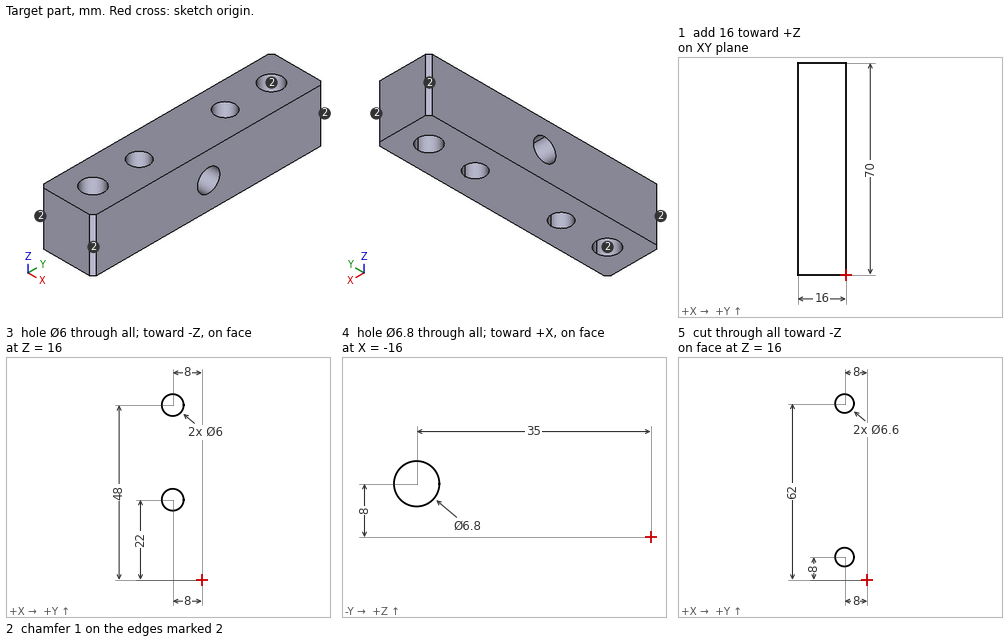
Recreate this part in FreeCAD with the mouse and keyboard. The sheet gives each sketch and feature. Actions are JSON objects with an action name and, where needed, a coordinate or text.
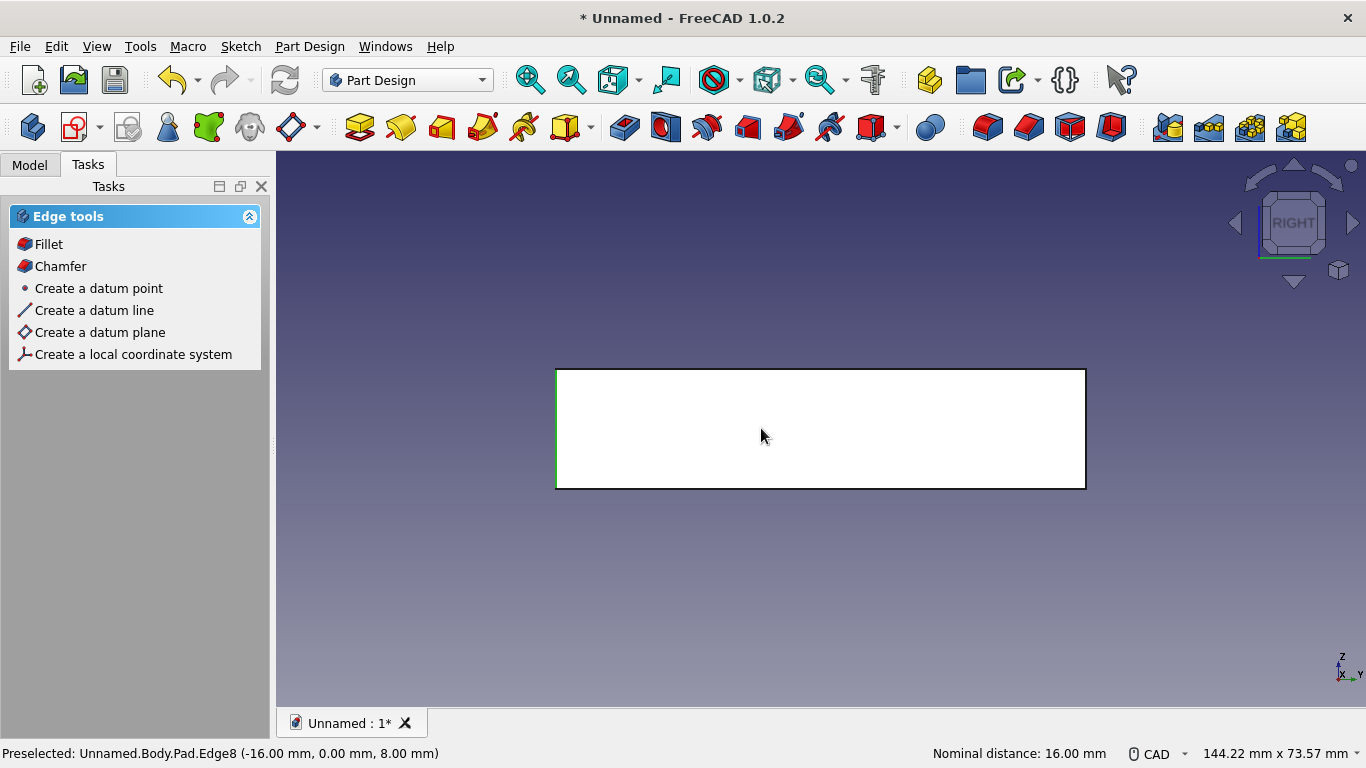
{"action": "left_click", "coordinate": [1086, 428], "text": "ctrl"}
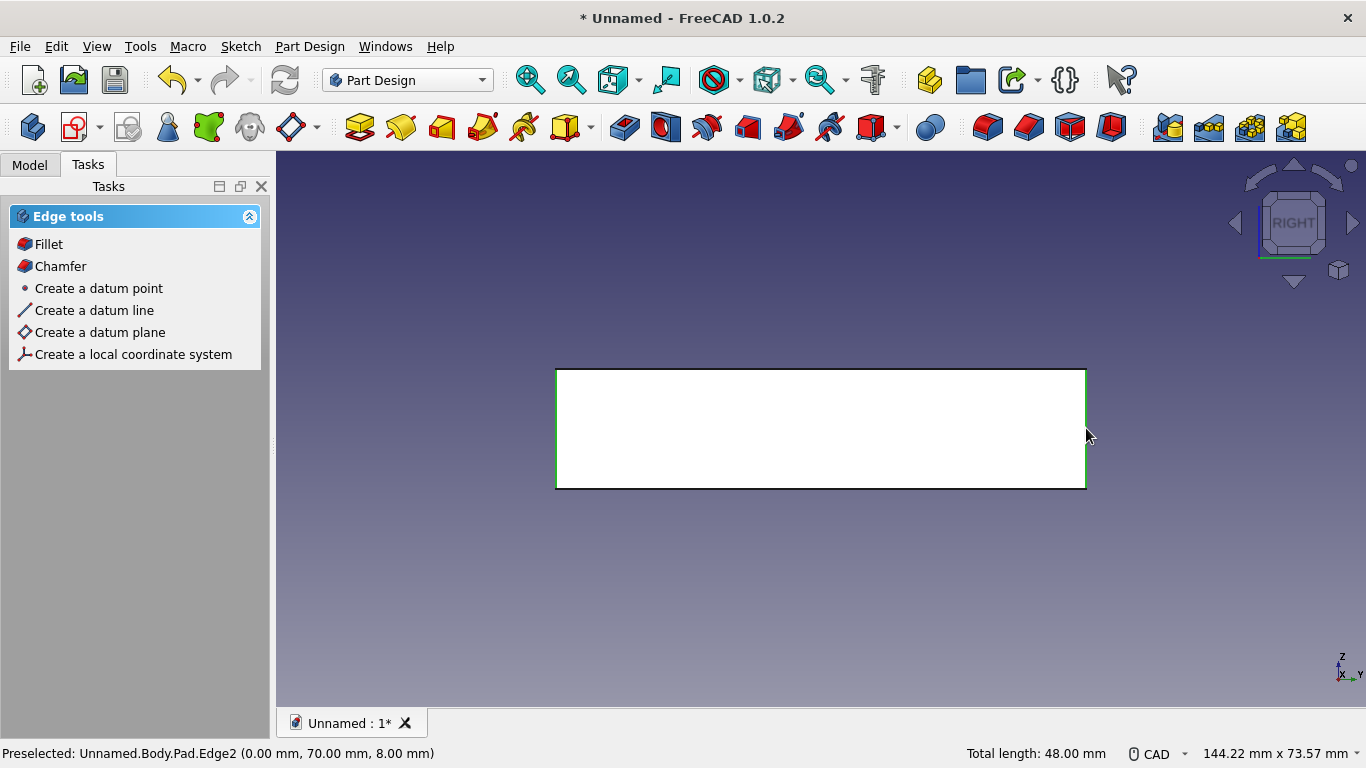
{"action": "key", "text": "5"}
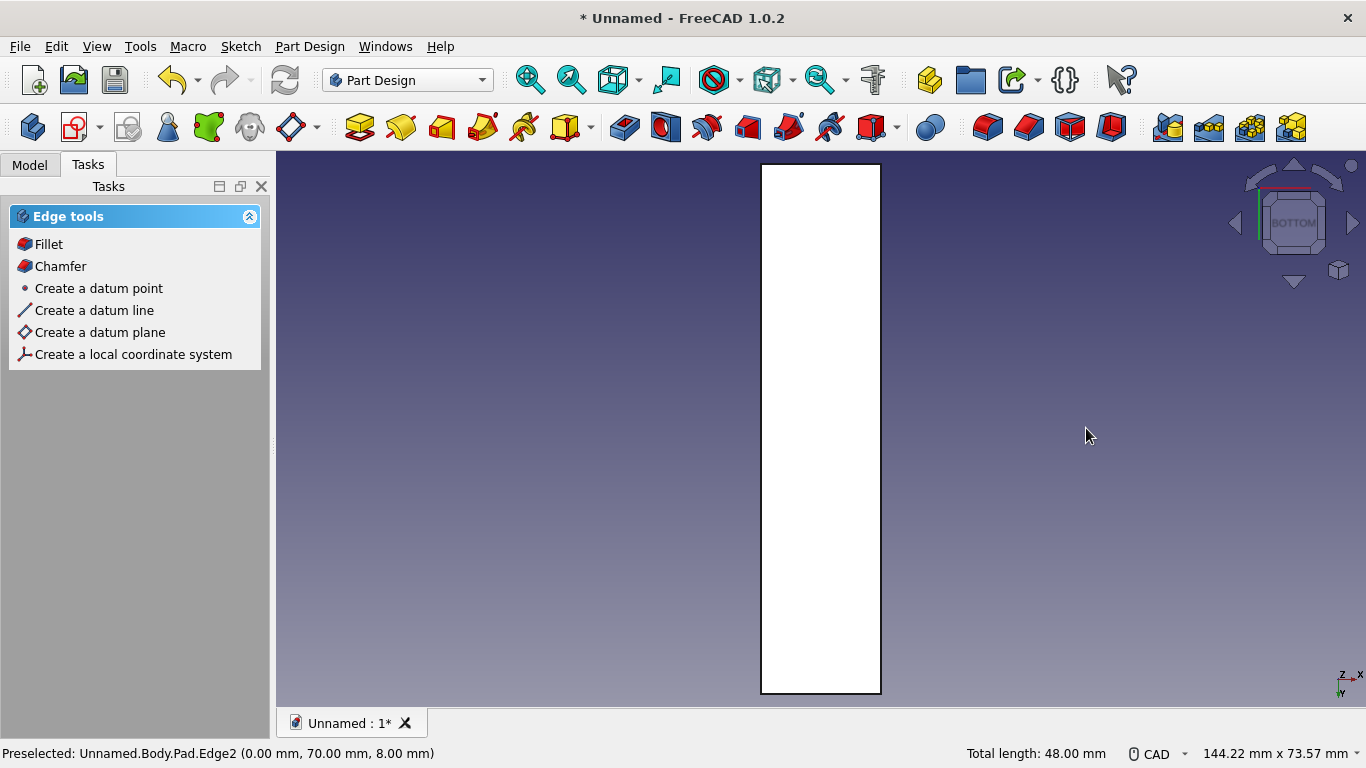
{"action": "key", "text": "4"}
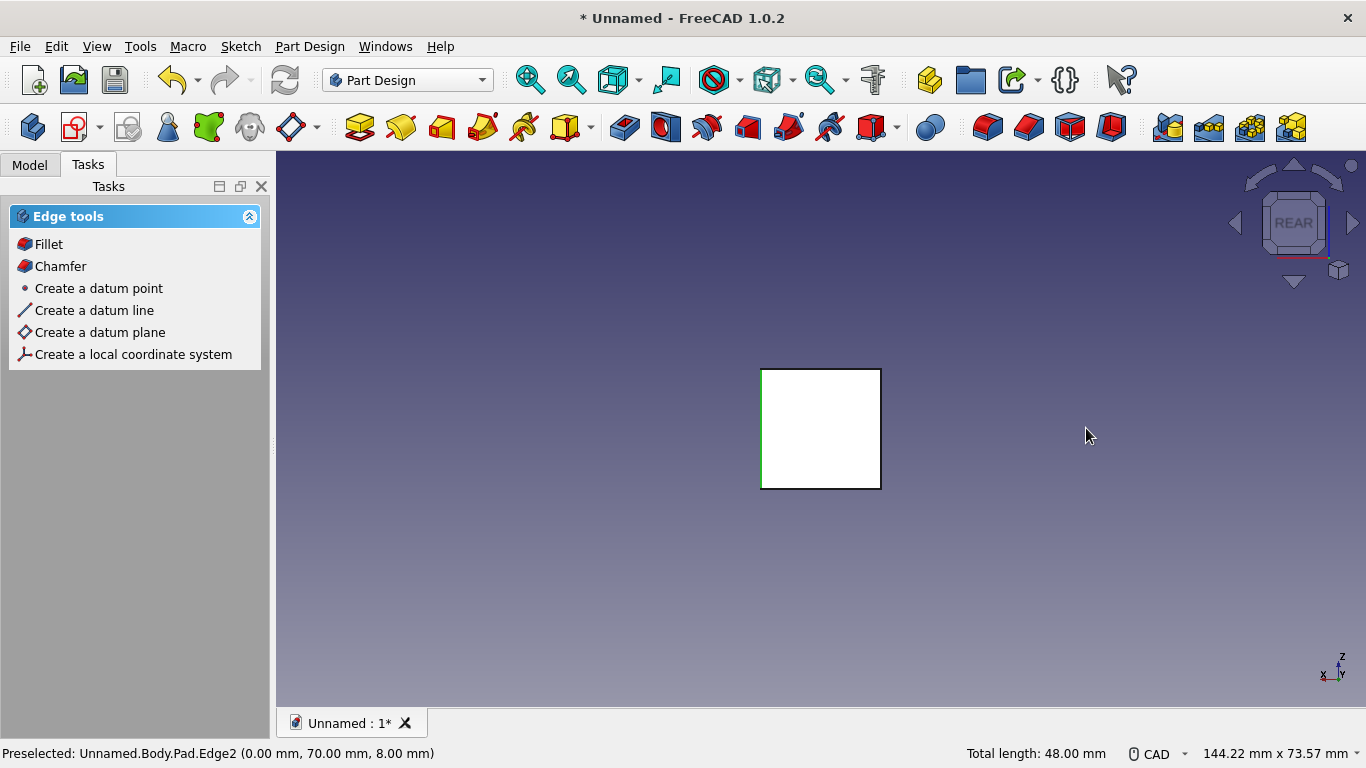
{"action": "left_click", "coordinate": [531, 80]}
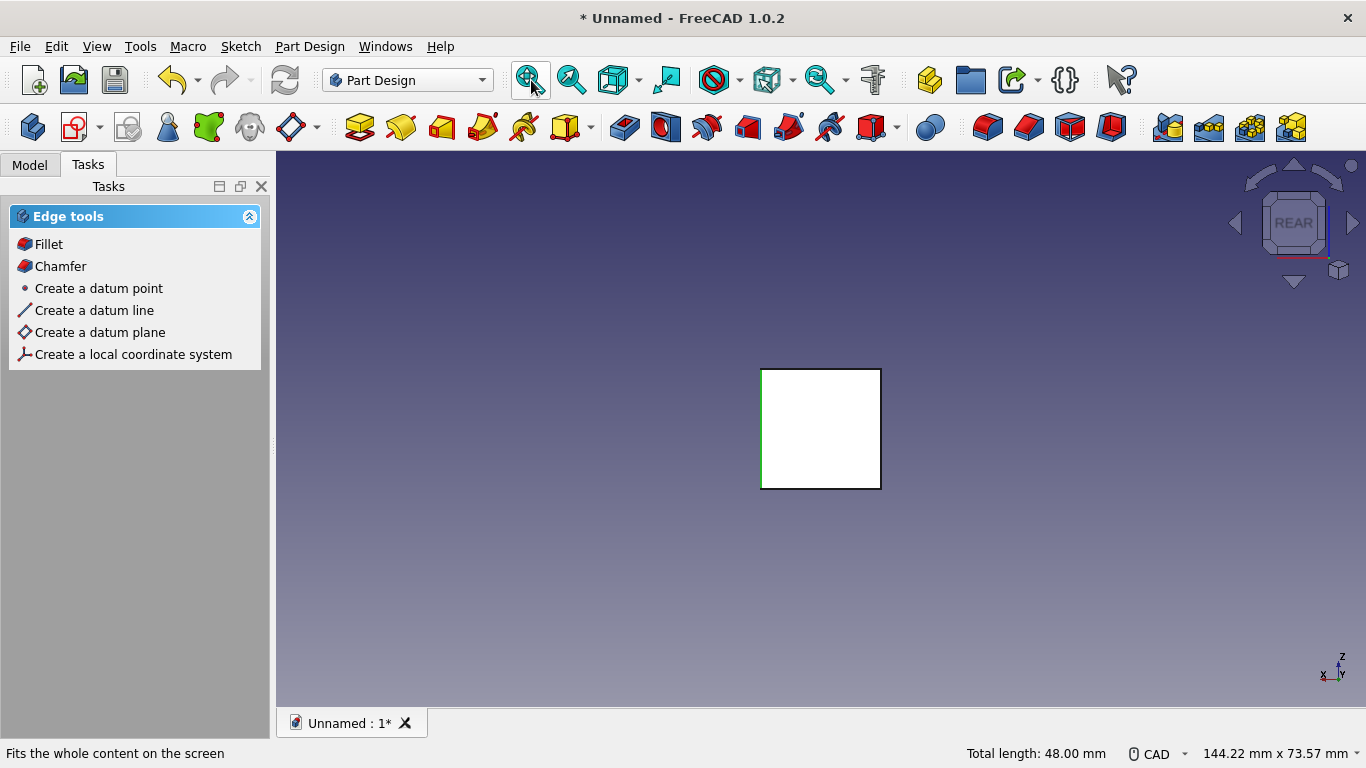
{"action": "left_click", "coordinate": [881, 428], "text": "ctrl"}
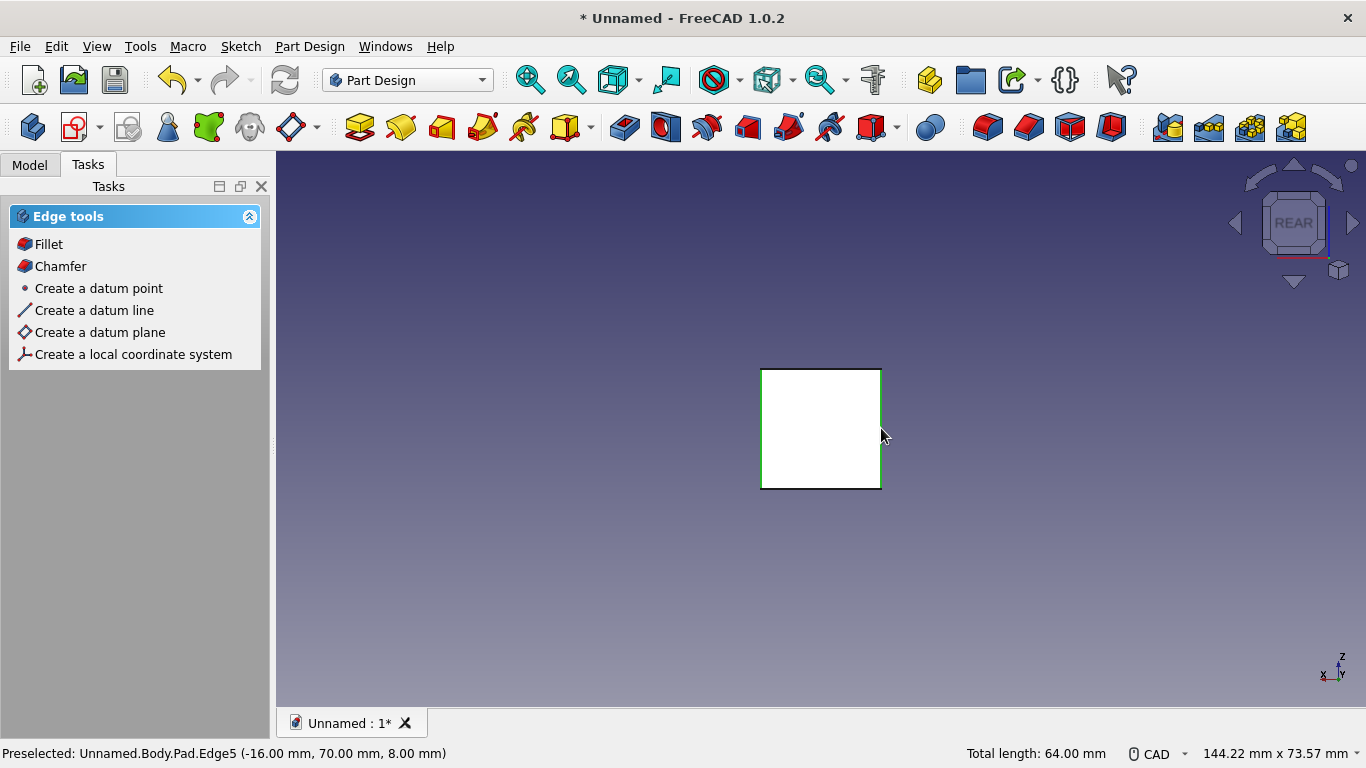
{"action": "left_click", "coordinate": [1029, 128]}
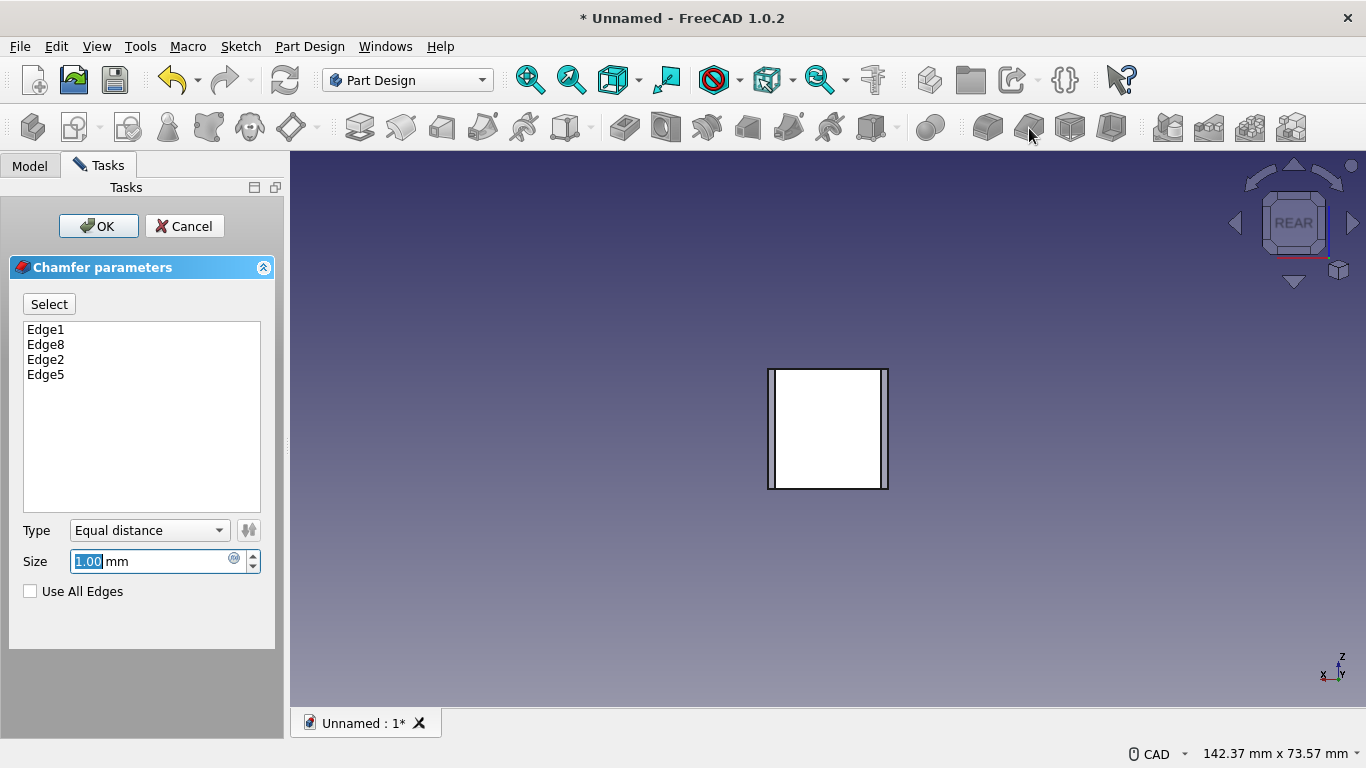
{"action": "type", "text": "1"}
{"action": "key", "text": "Tab"}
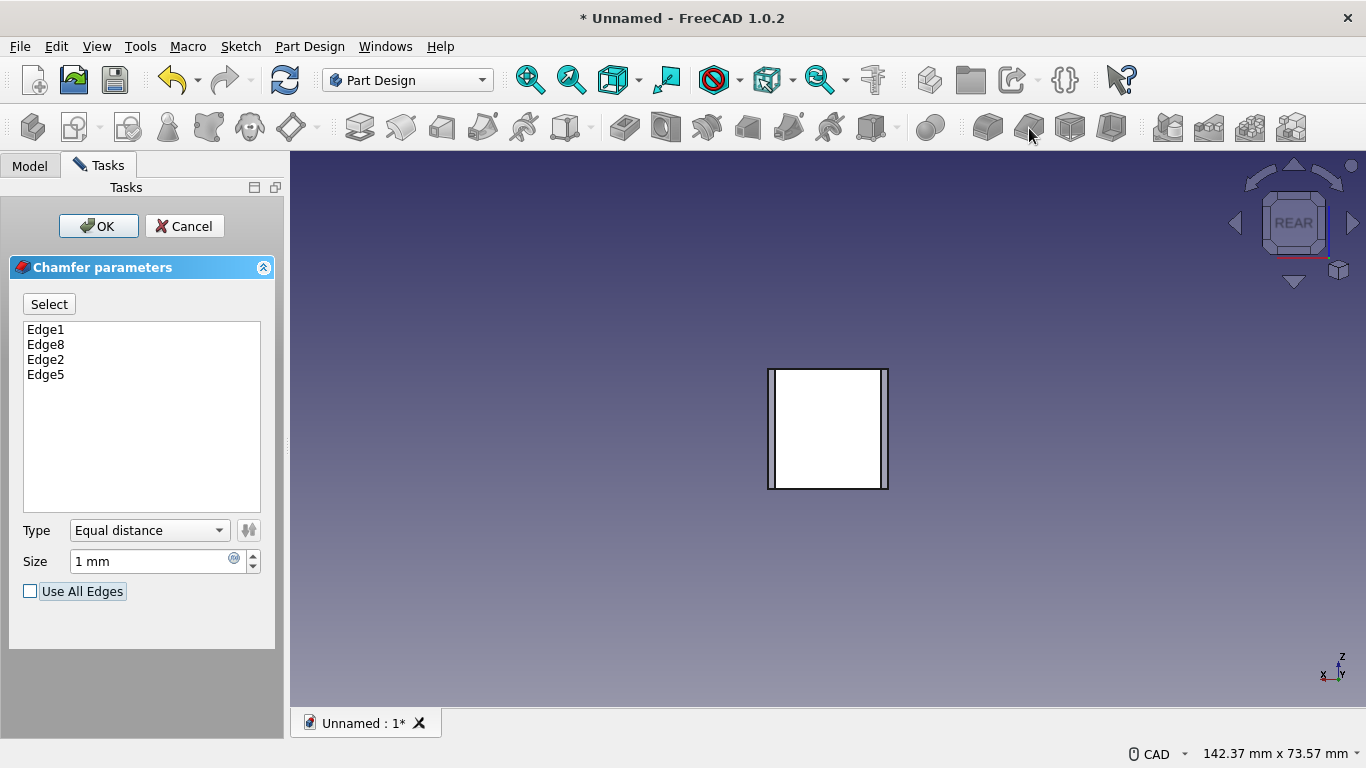
{"action": "left_click", "coordinate": [99, 226]}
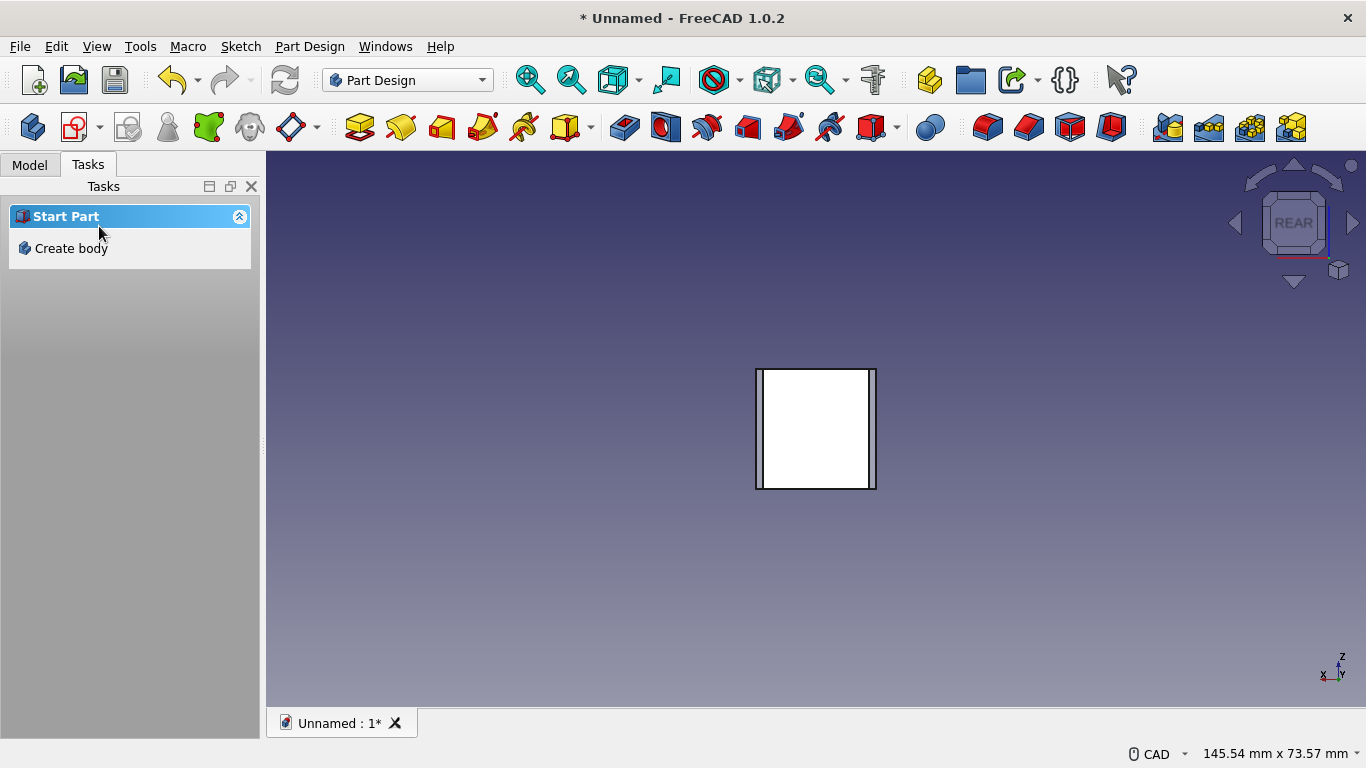
{"action": "left_click", "coordinate": [531, 80]}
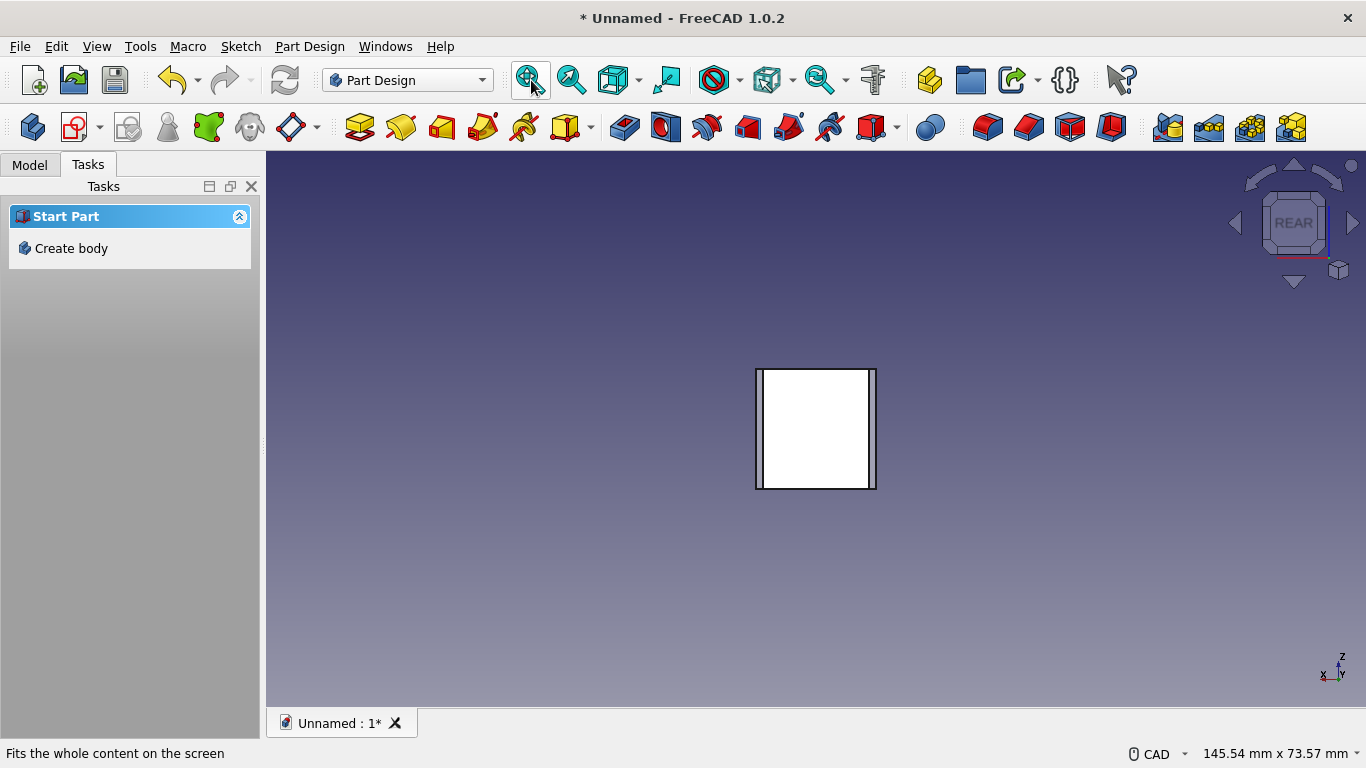
{"action": "key", "text": "0"}